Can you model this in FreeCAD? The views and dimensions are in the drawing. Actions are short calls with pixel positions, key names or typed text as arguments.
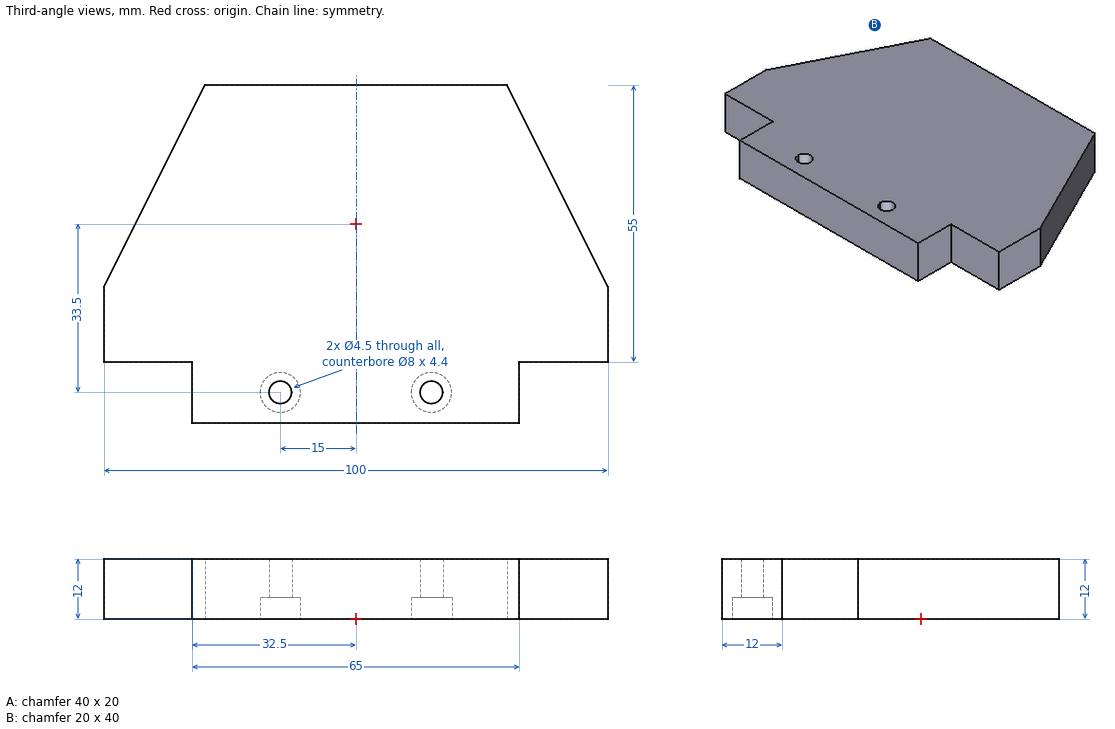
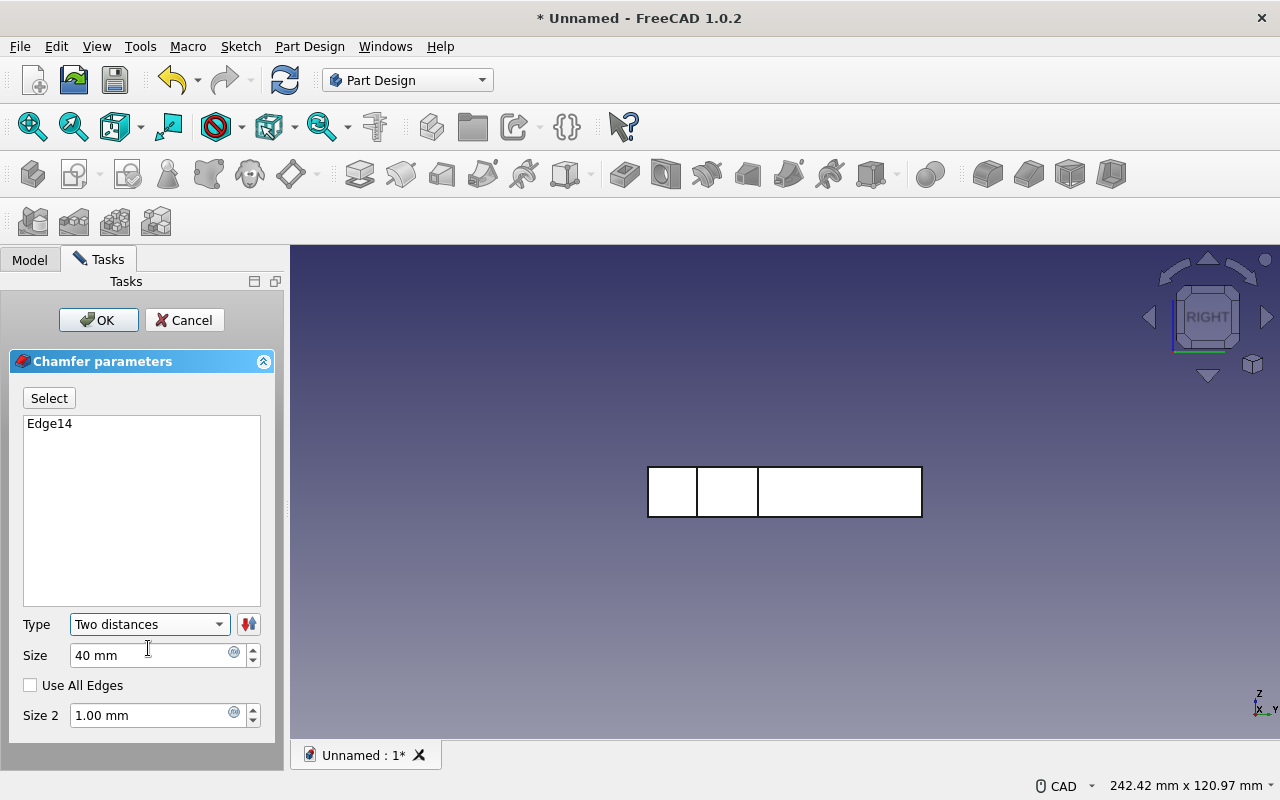
triple_click(158, 716)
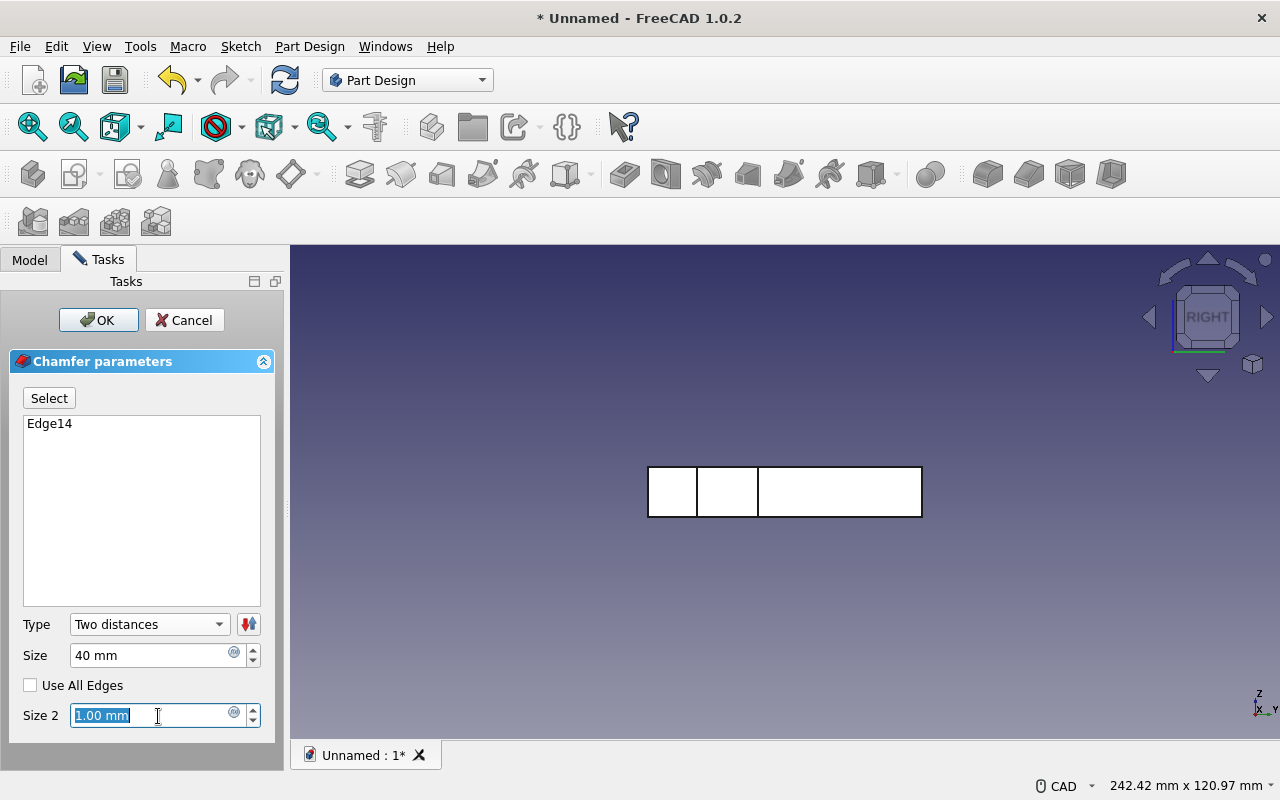
text(20)
key(Tab)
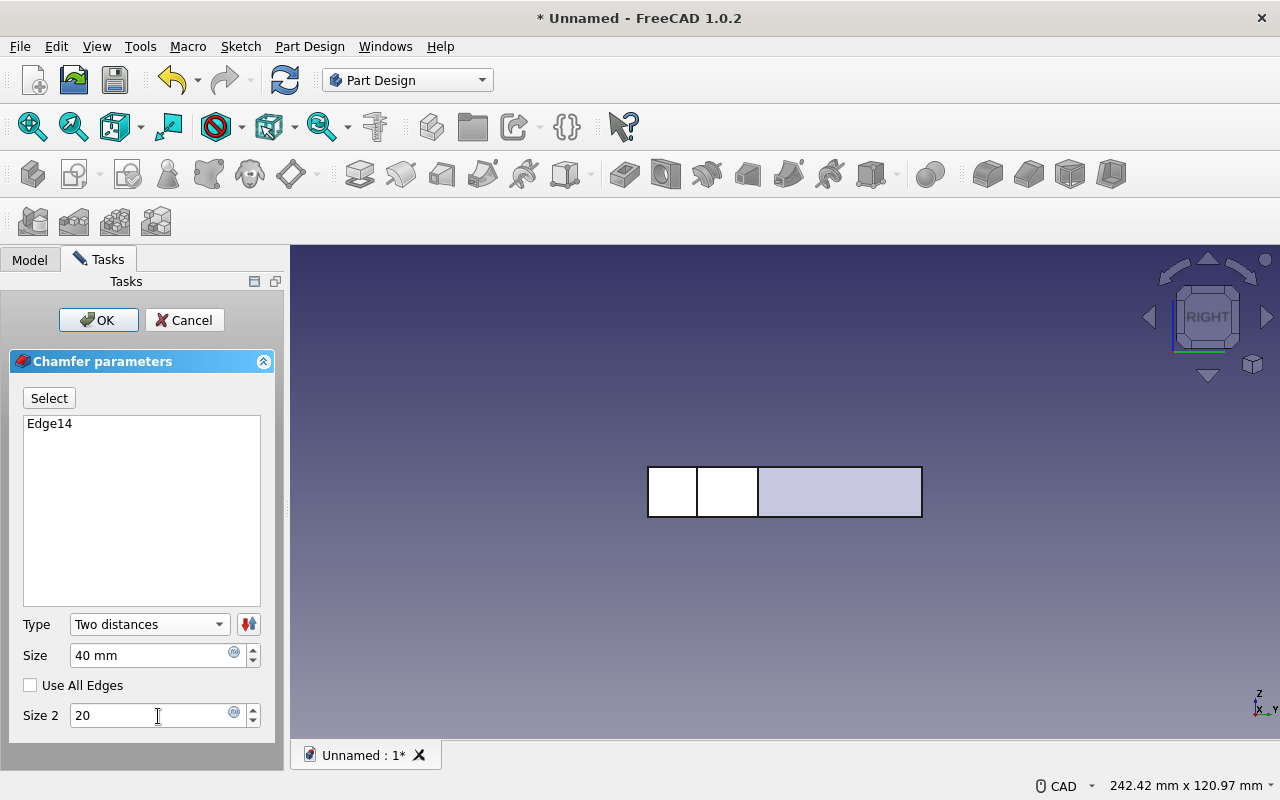
click(99, 320)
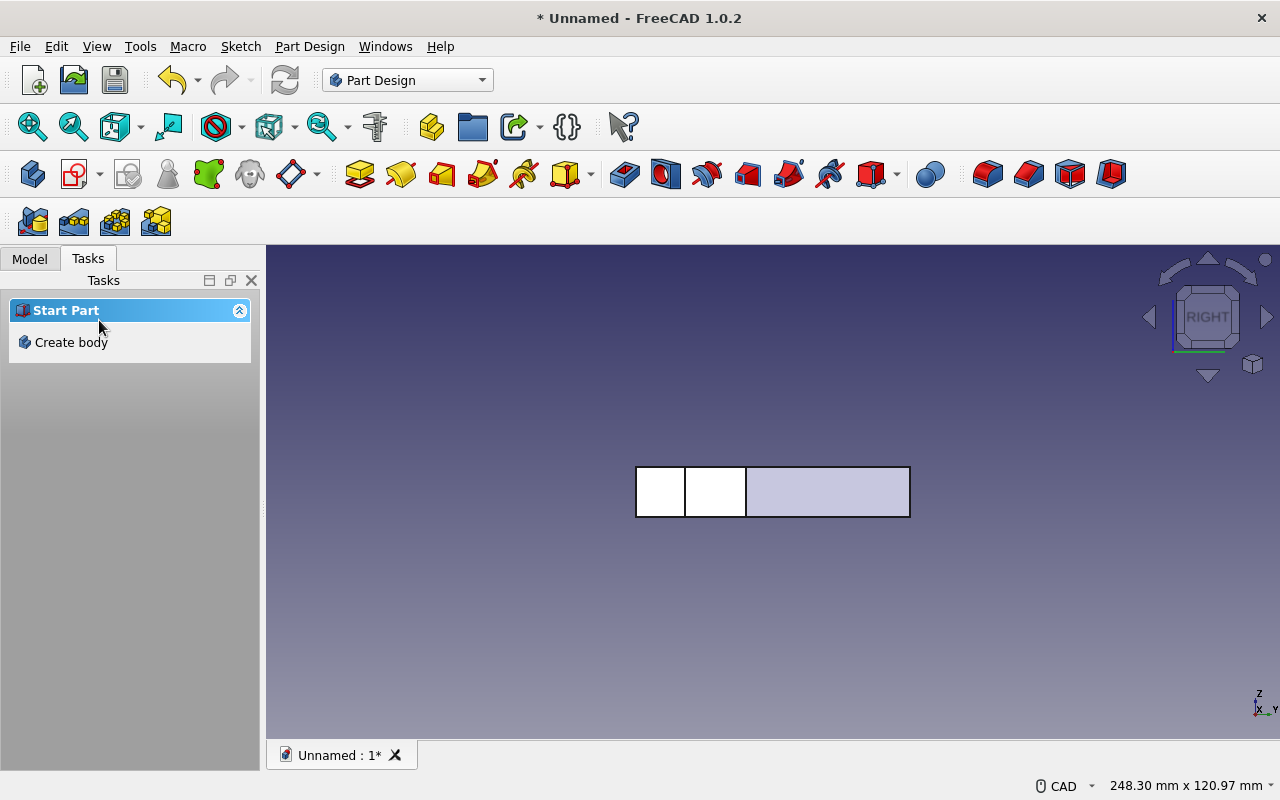
click(33, 128)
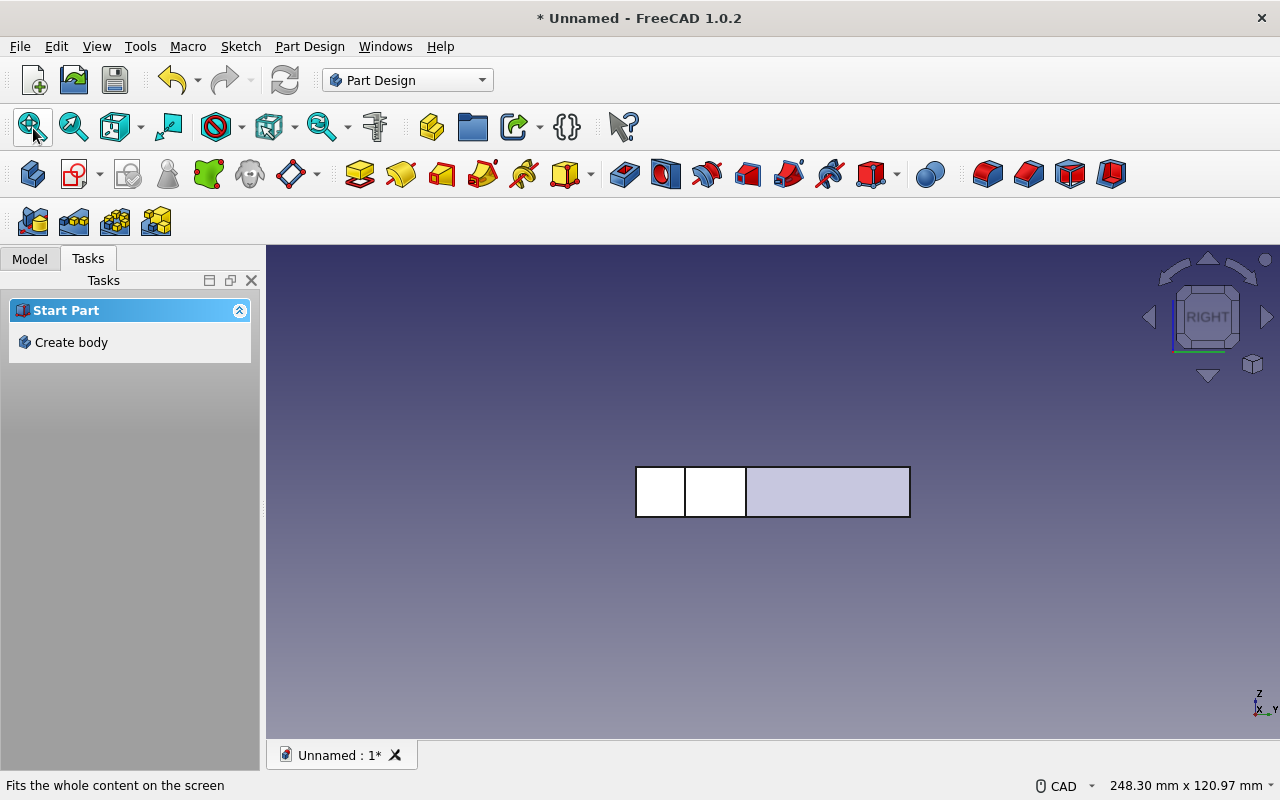
key(0)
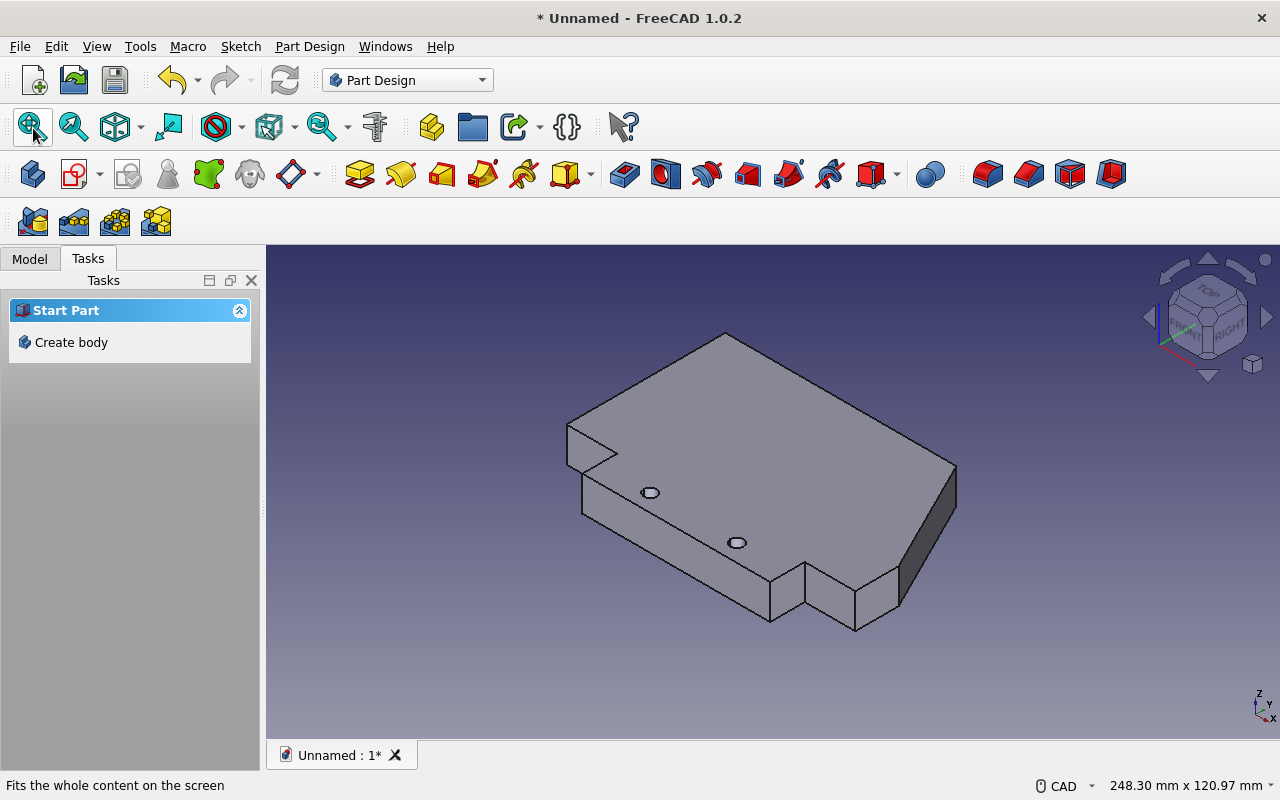
key(2)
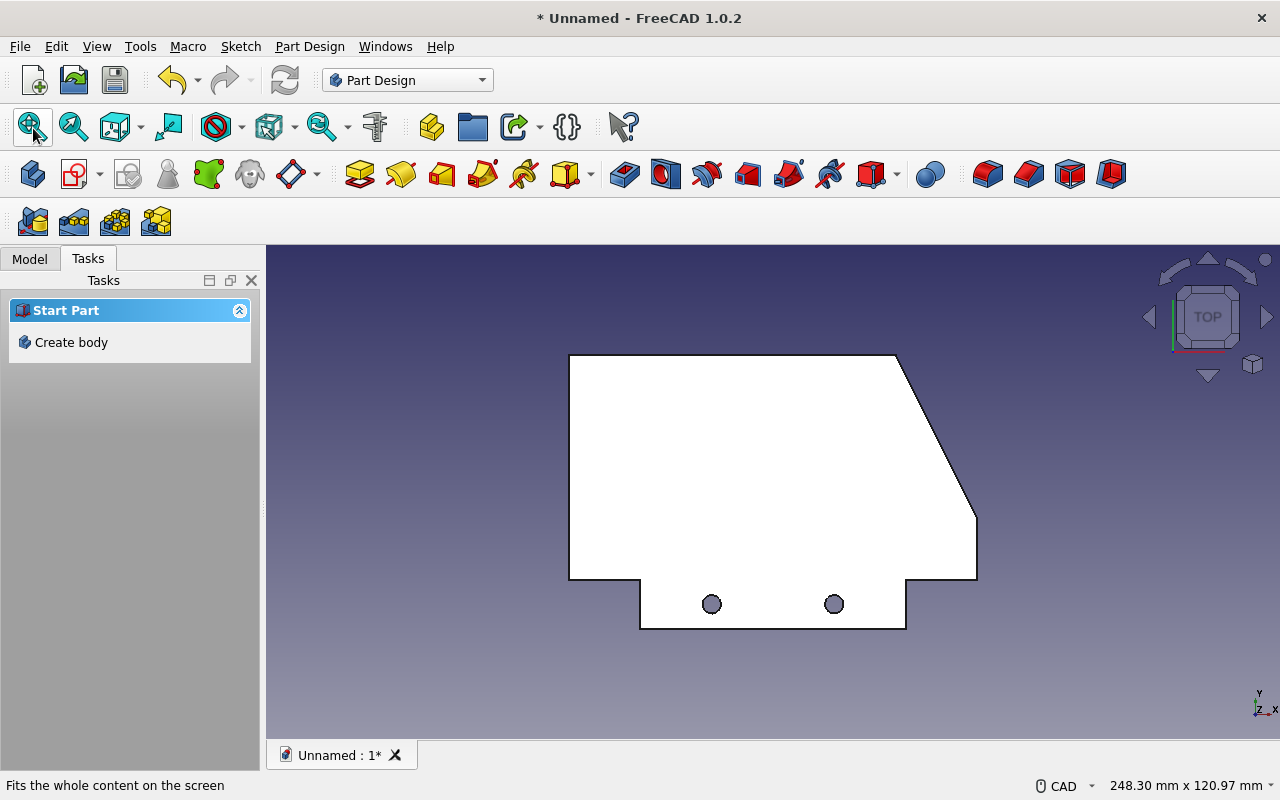
key(1)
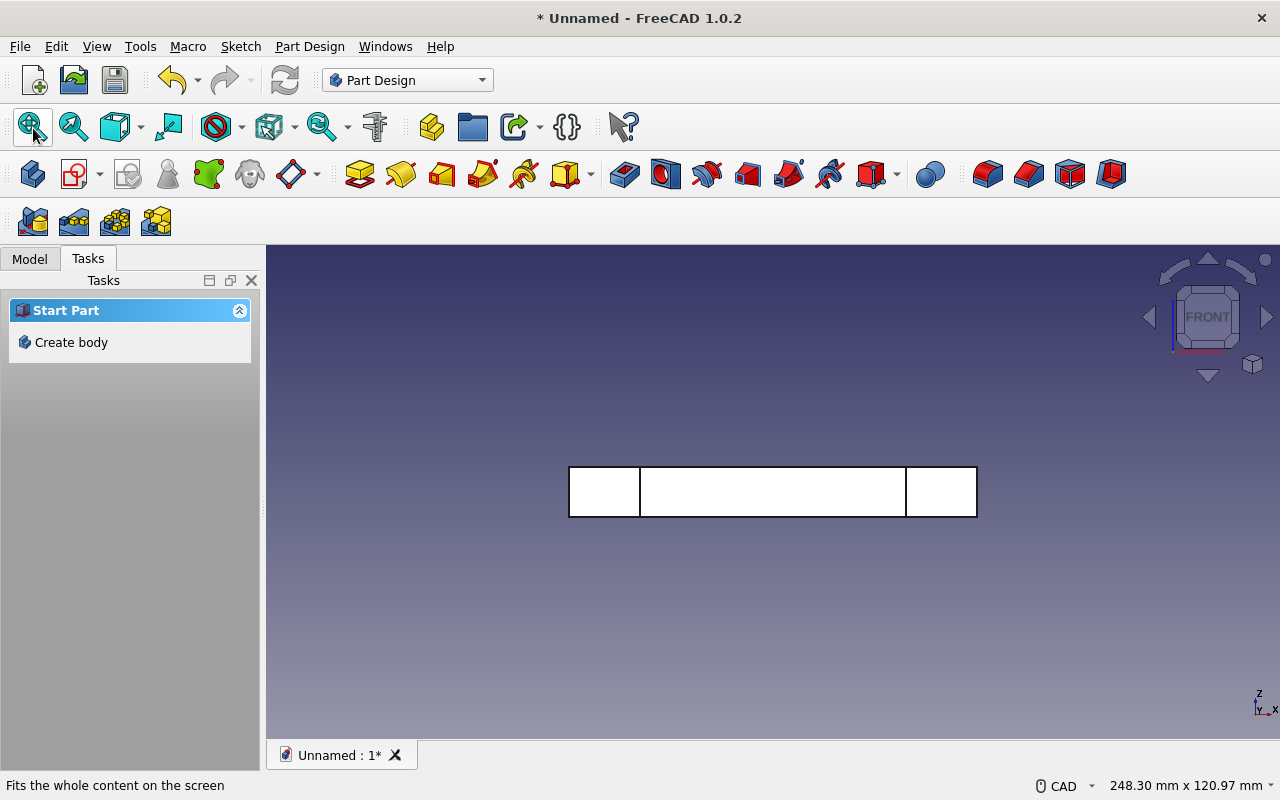
click(33, 128)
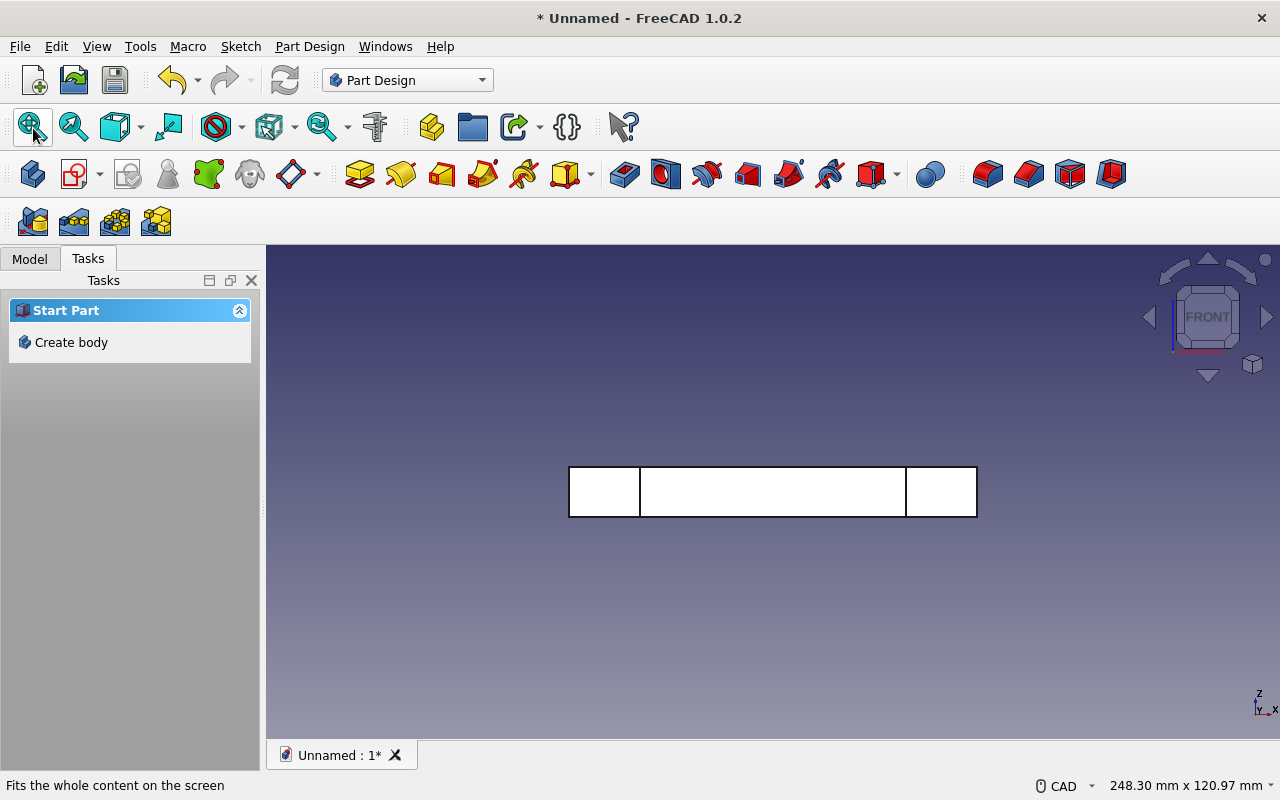
key(3)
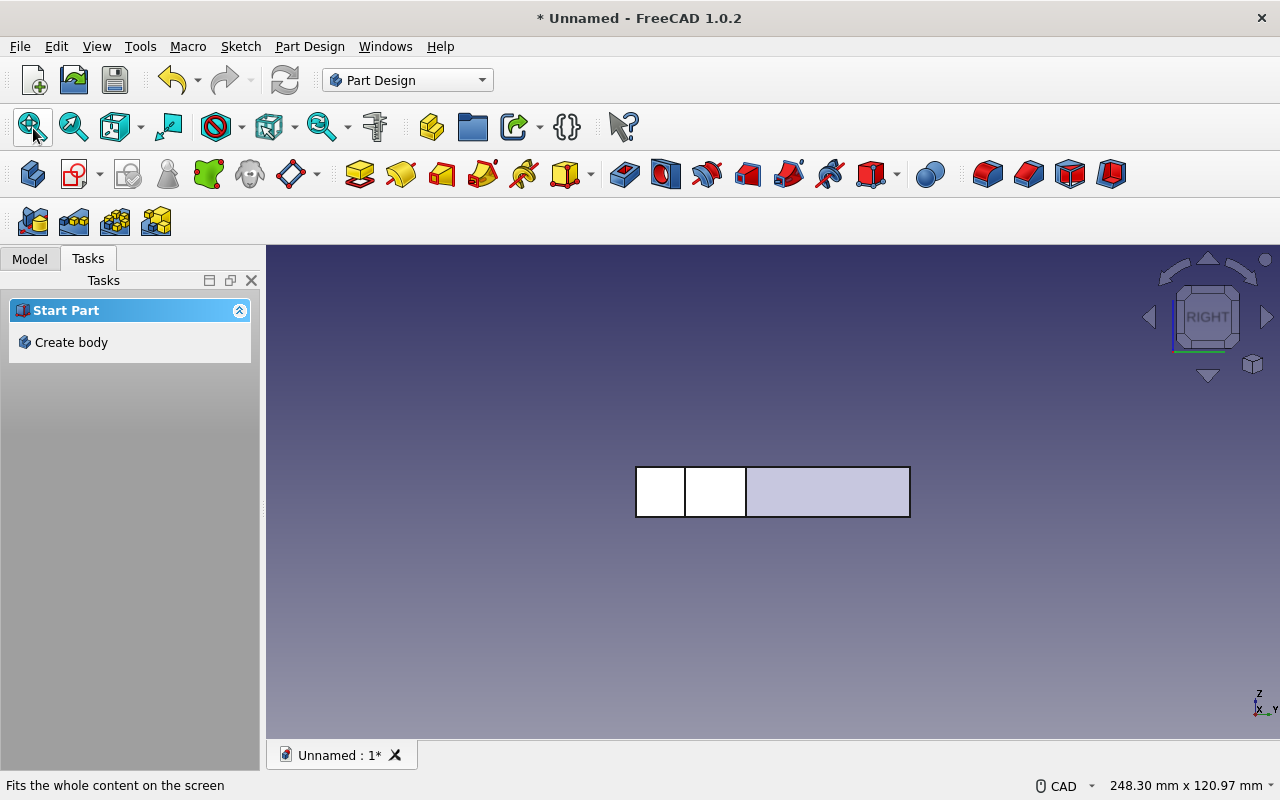
click(33, 128)